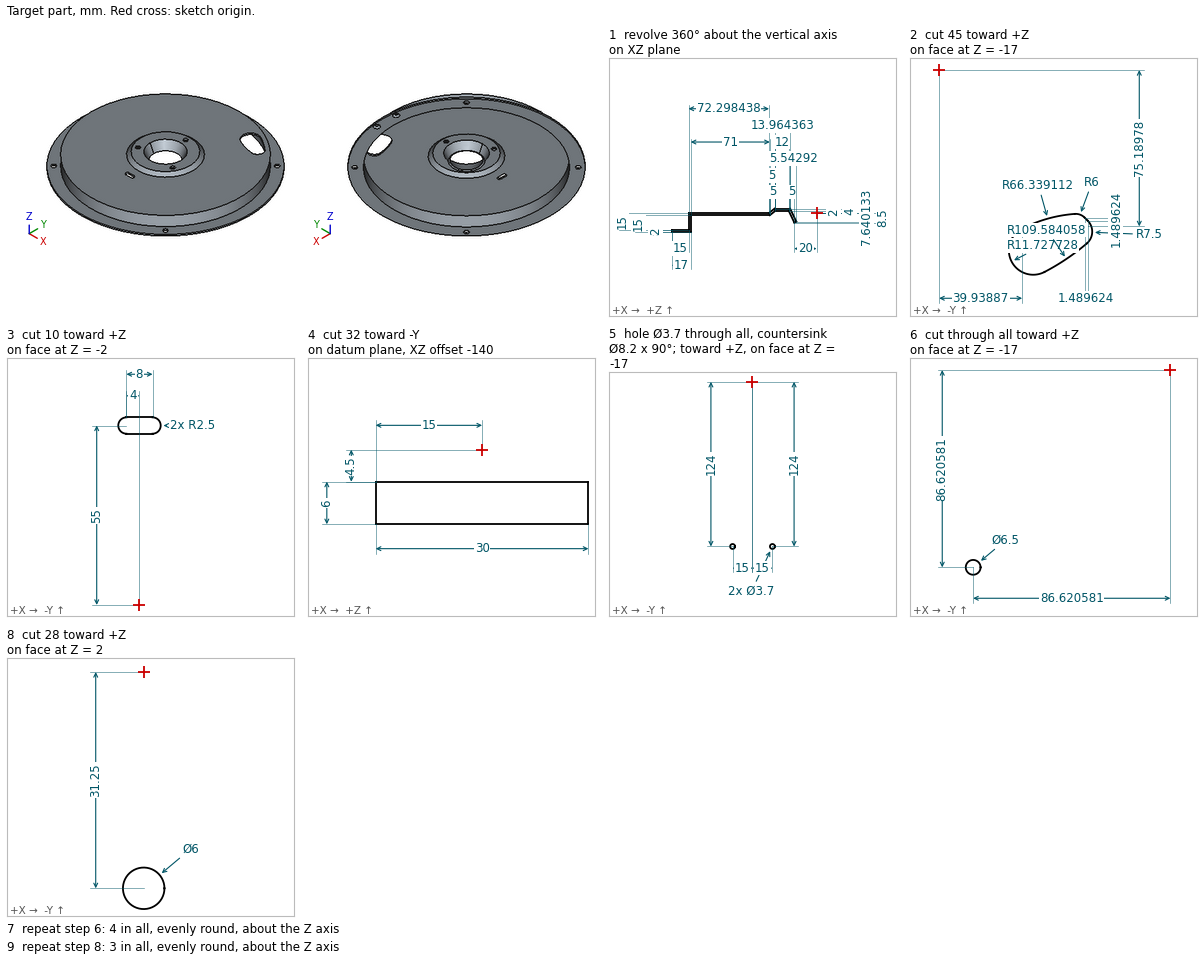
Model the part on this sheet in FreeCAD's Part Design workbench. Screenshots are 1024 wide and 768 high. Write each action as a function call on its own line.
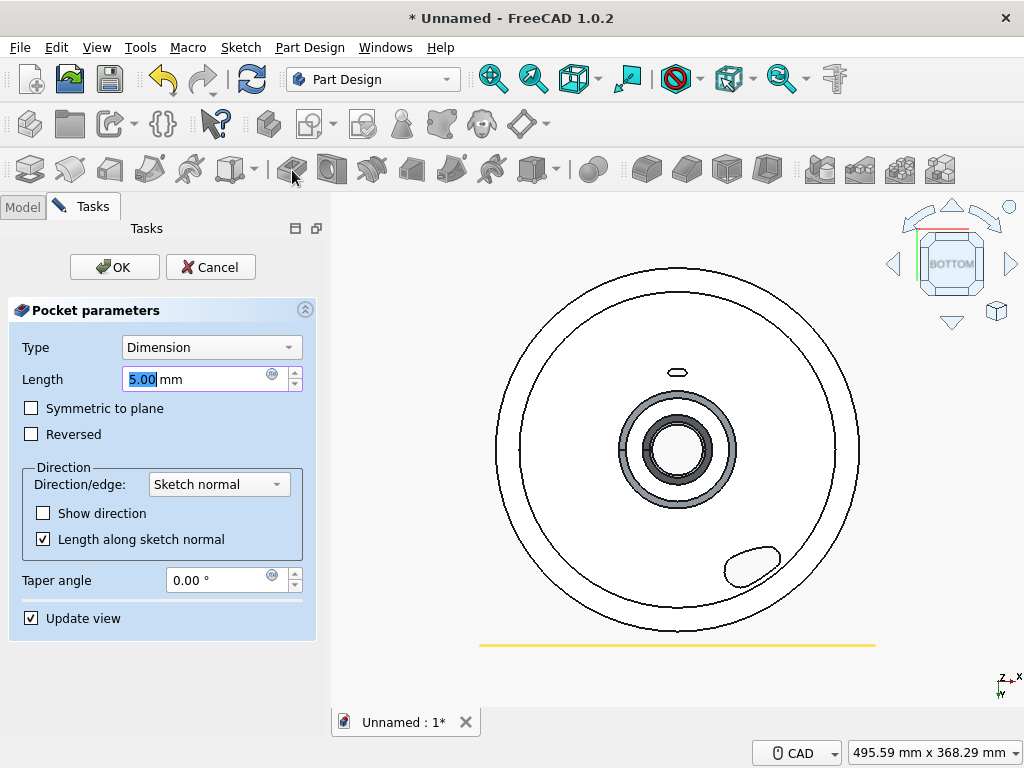
text(32)
key(Tab)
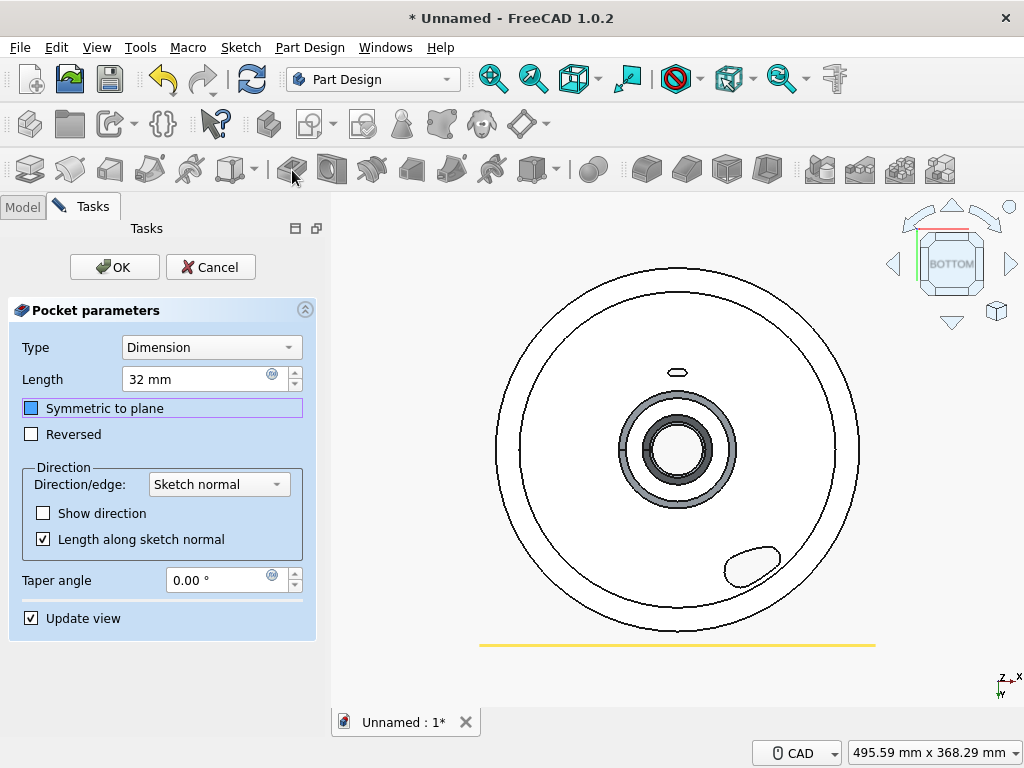
click(30, 434)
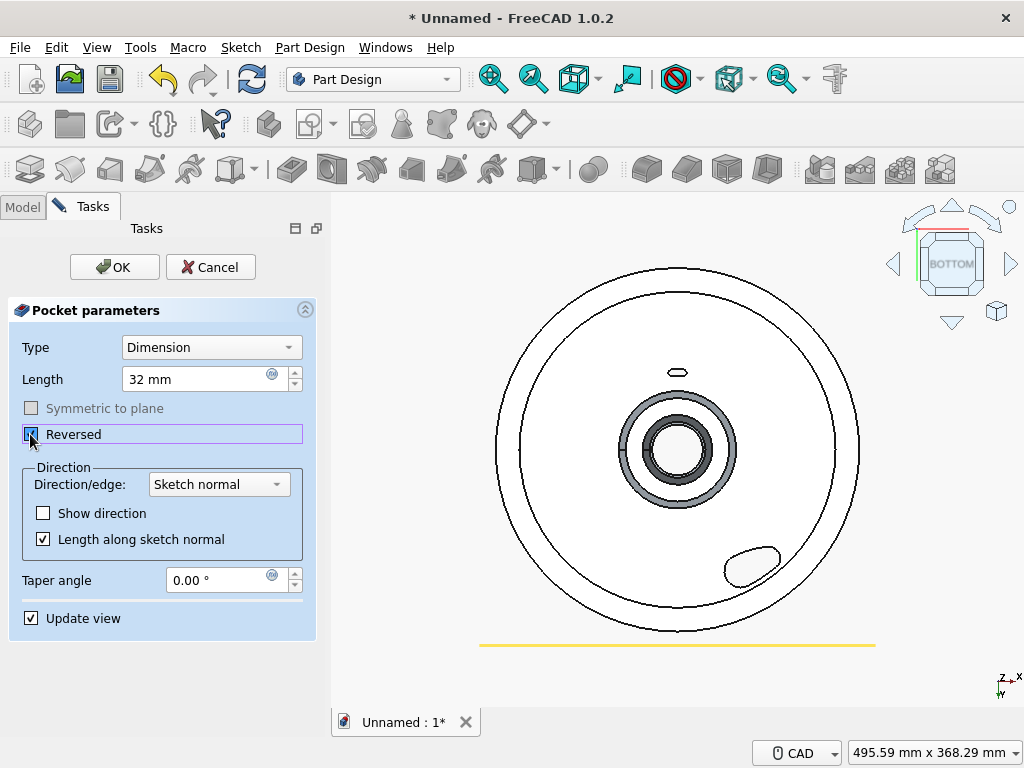
click(115, 267)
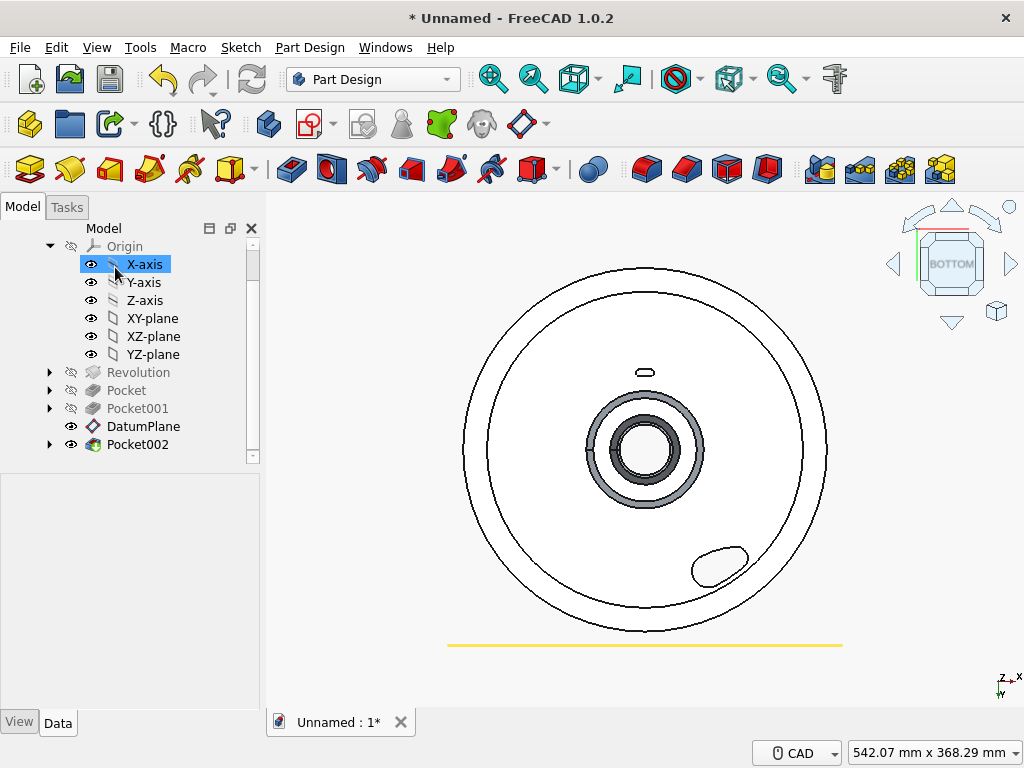
click(116, 426)
key(space)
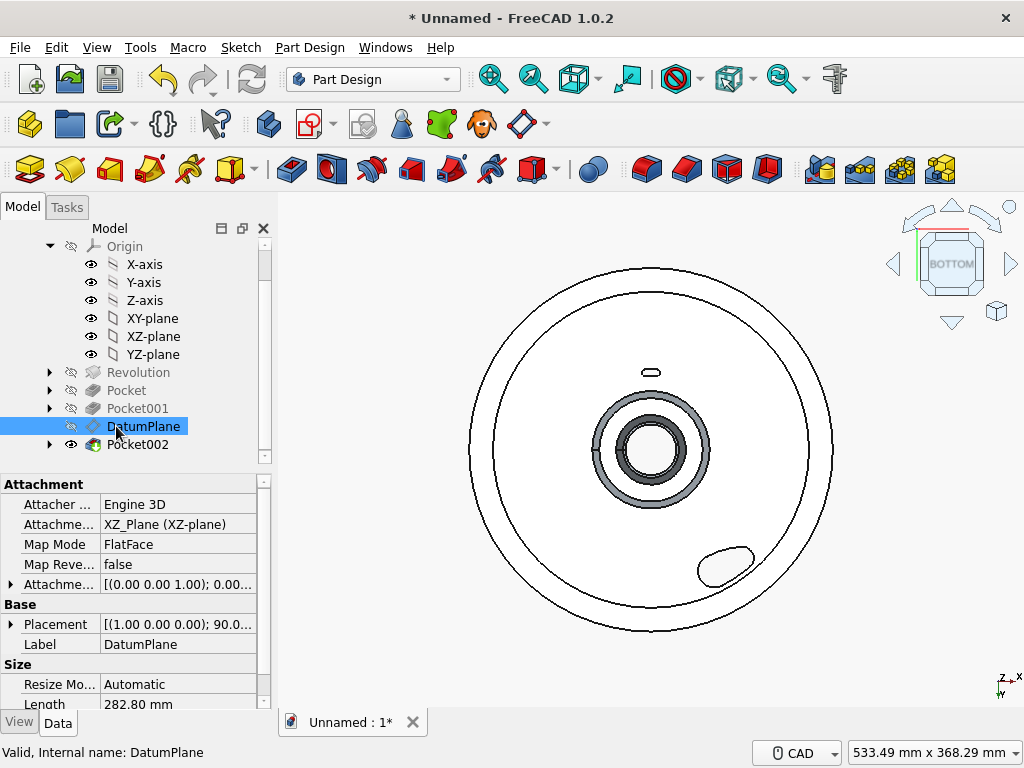
click(599, 293)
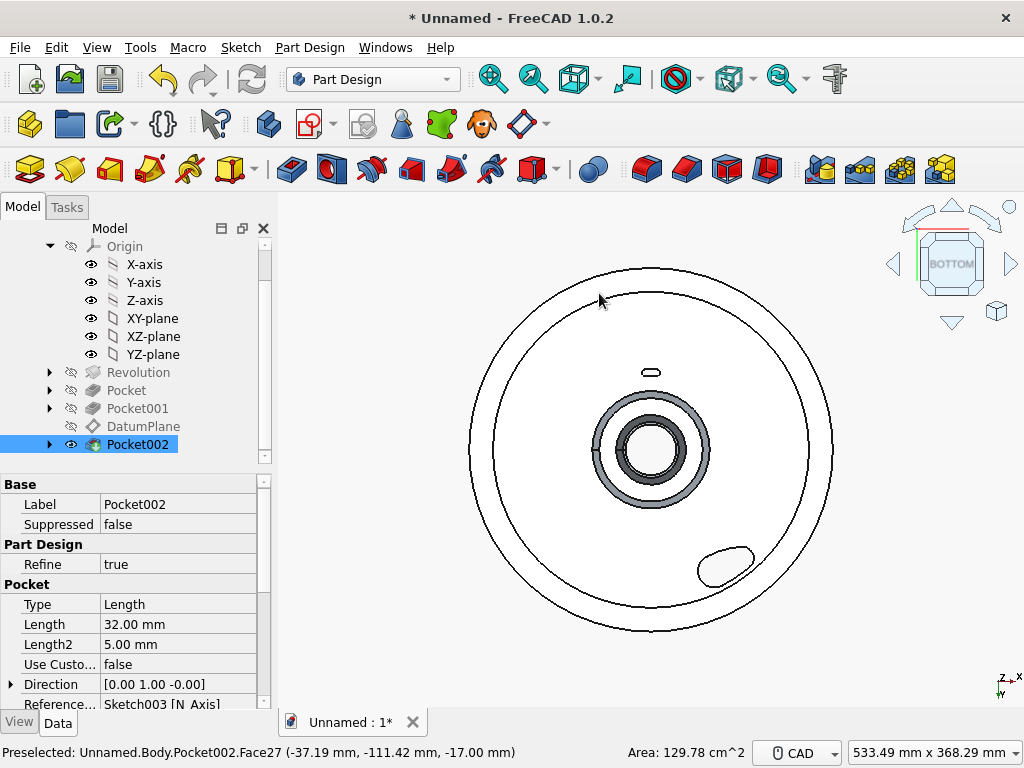
click(310, 124)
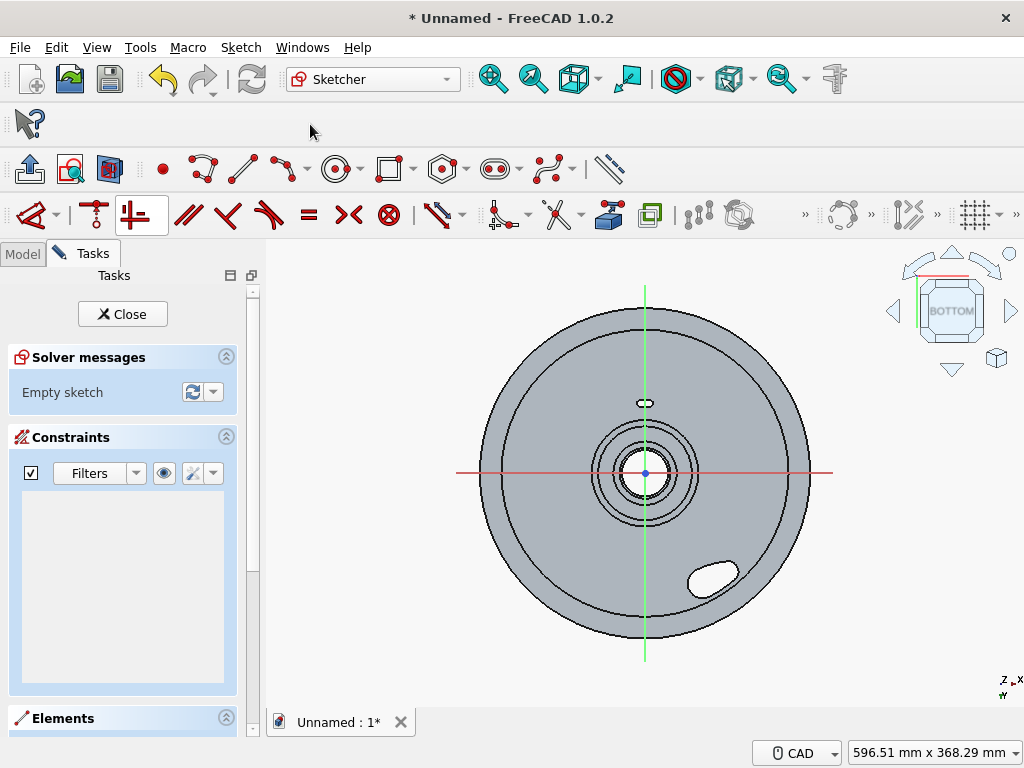
scroll(654, 651, up, 11)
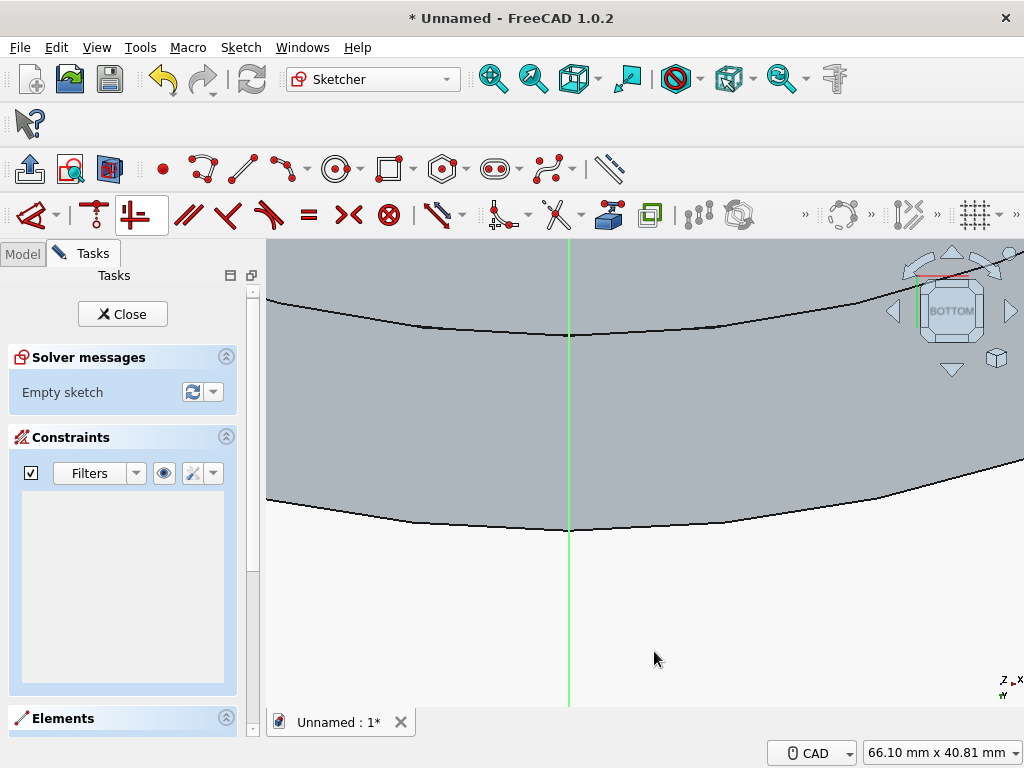
click(336, 170)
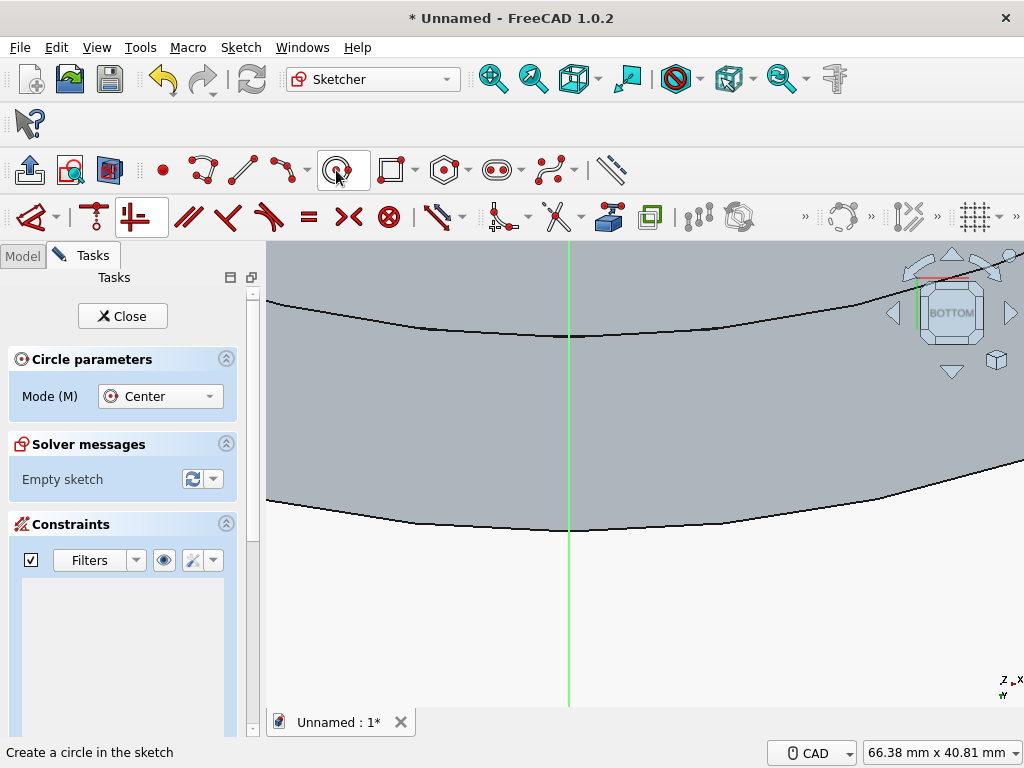
click(740, 463)
click(755, 448)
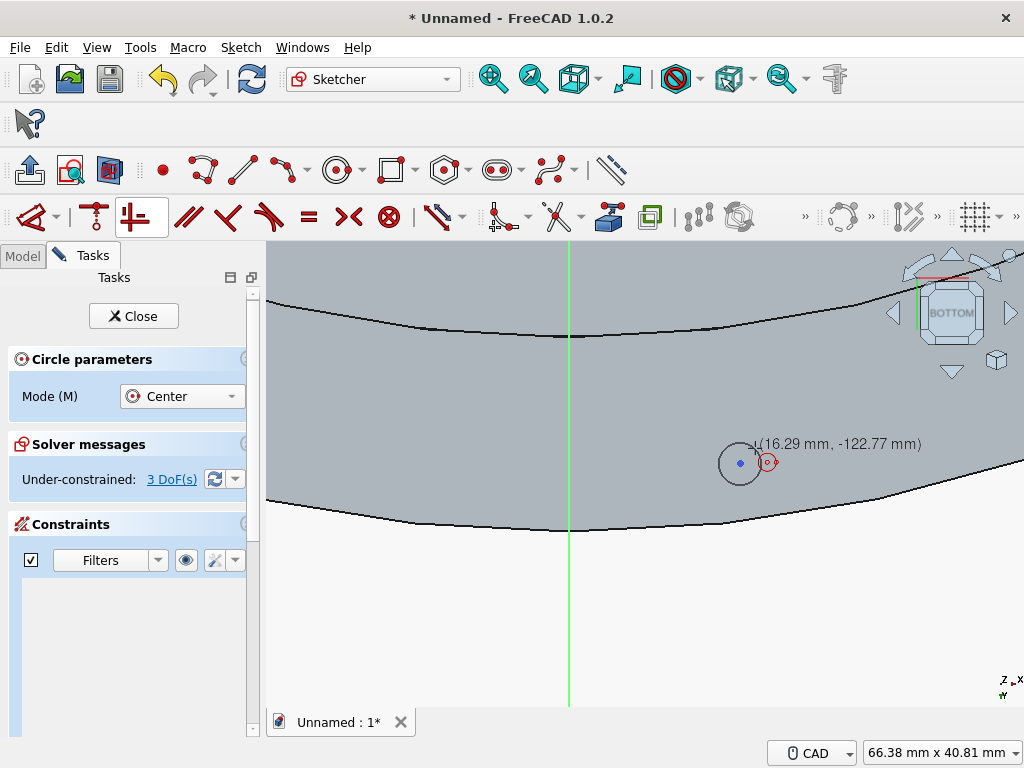
click(398, 463)
click(413, 448)
key(Escape)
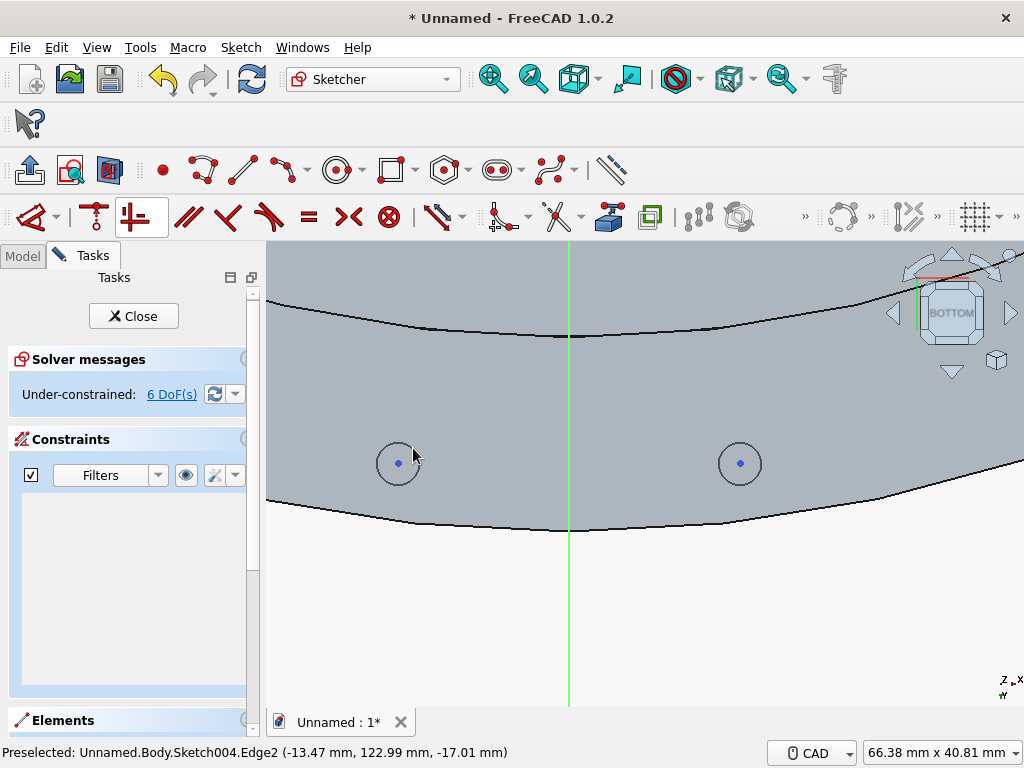
click(755, 449)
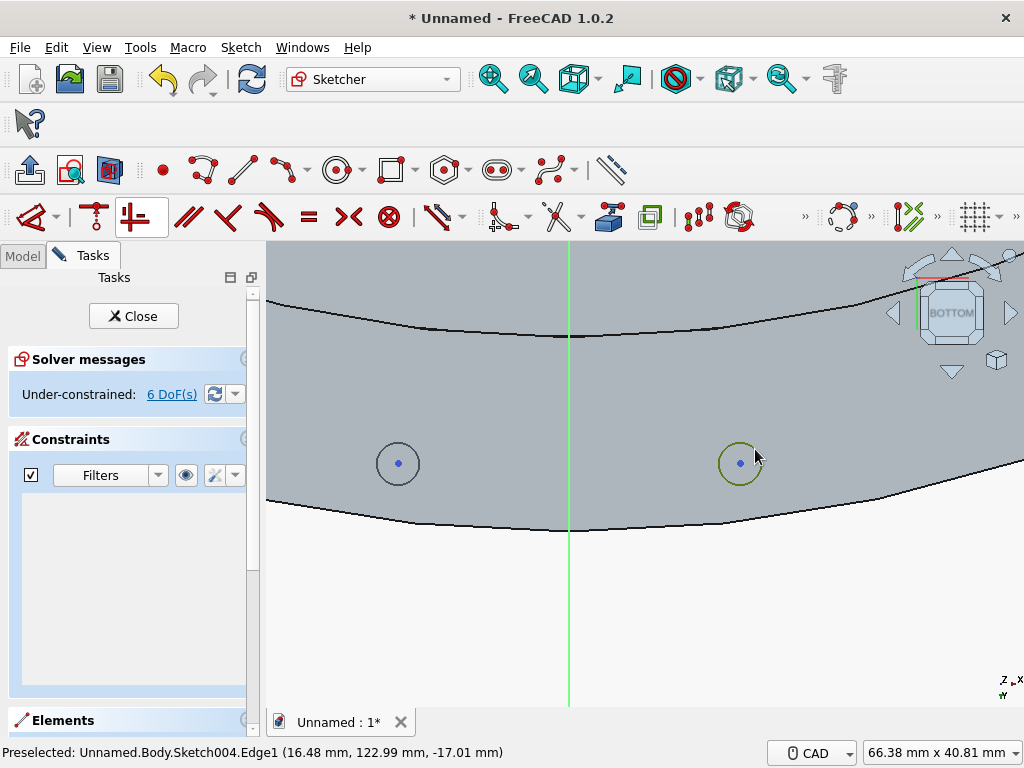
click(413, 449)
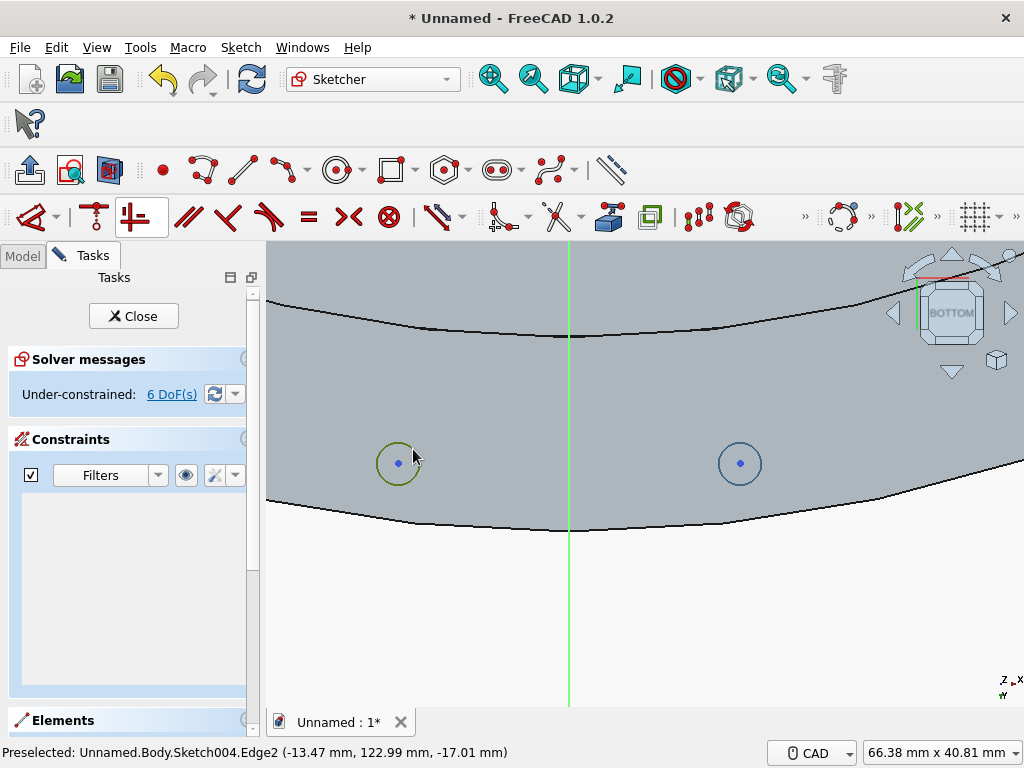
click(310, 218)